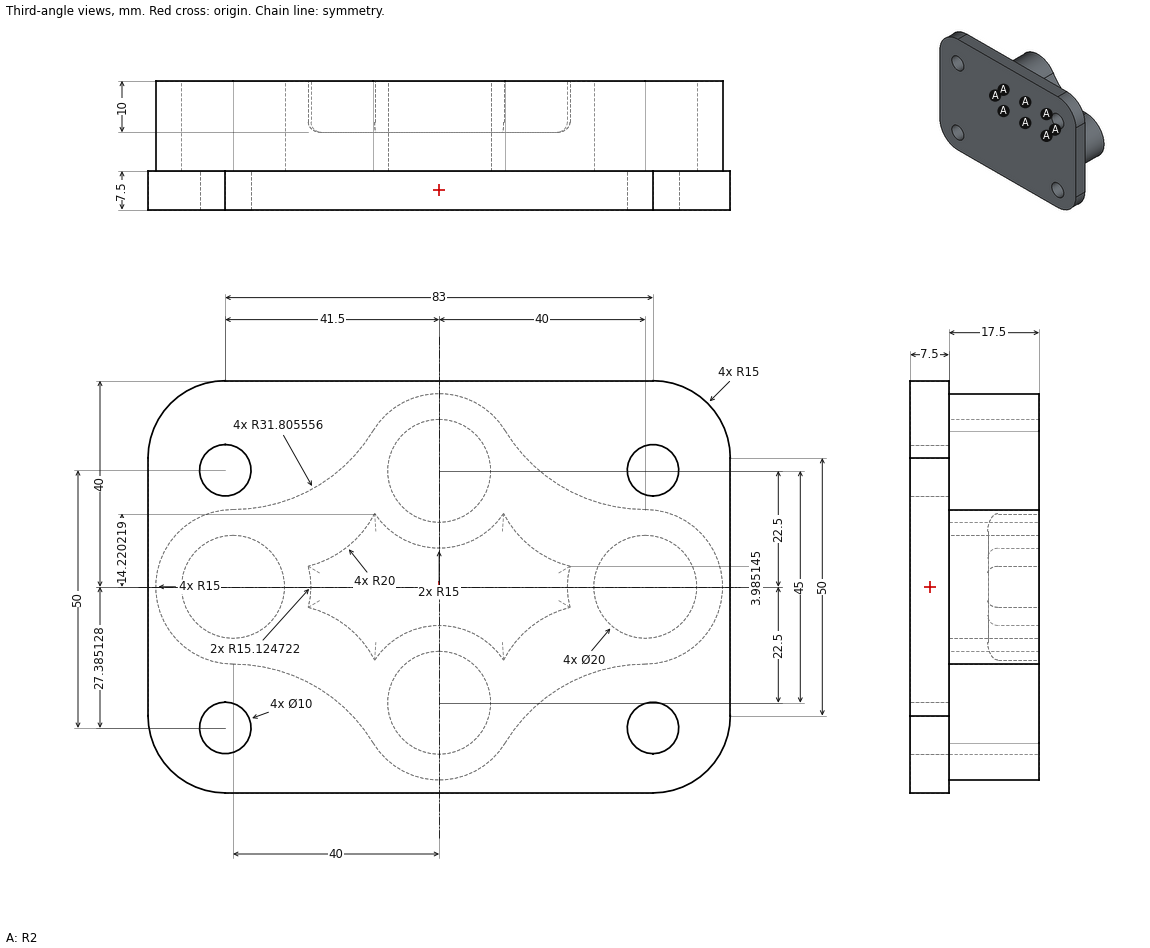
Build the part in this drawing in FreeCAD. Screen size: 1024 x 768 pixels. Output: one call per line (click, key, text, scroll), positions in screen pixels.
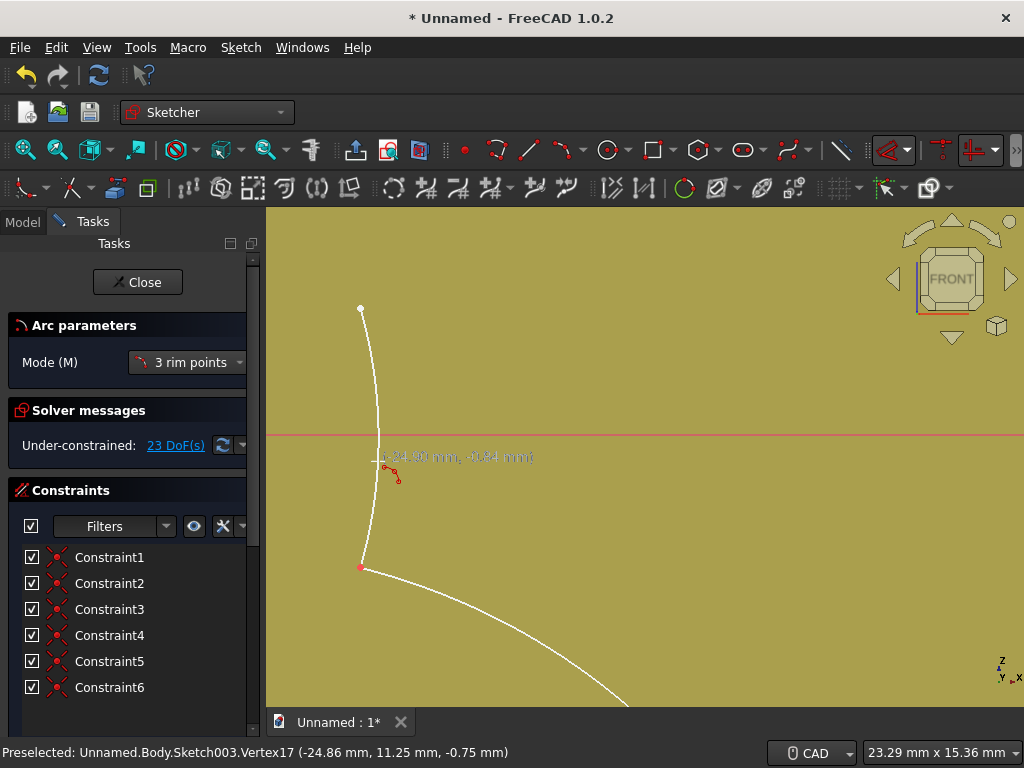
scroll(376, 464, down, 7)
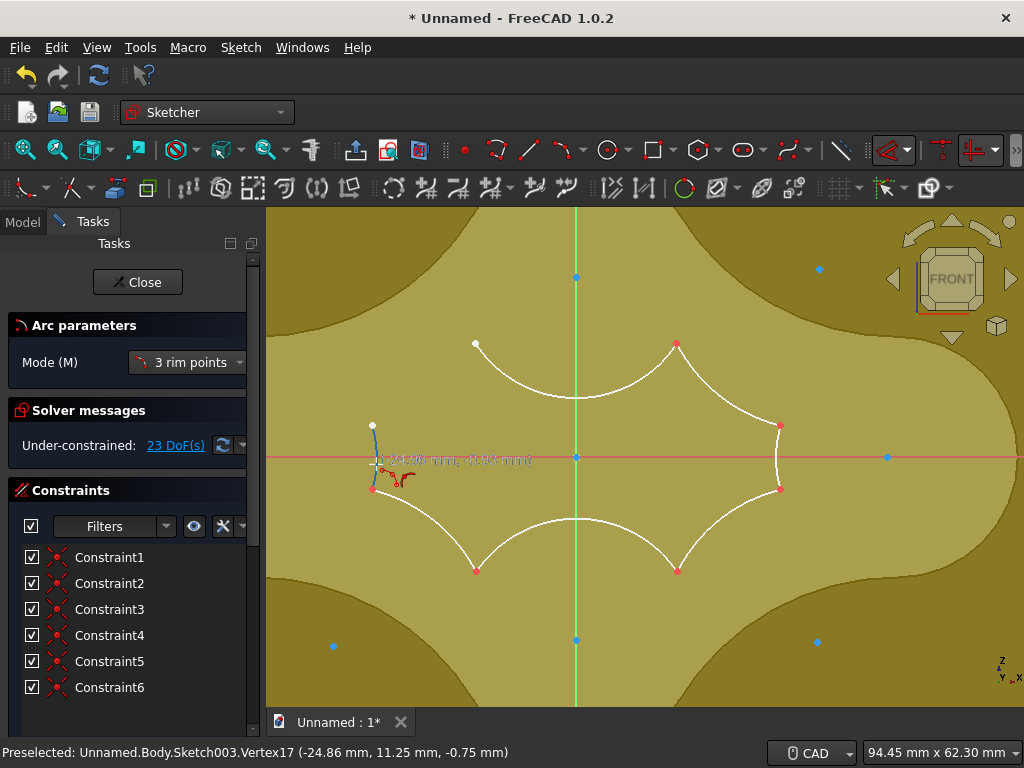
click(372, 426)
click(476, 344)
click(433, 395)
key(Escape)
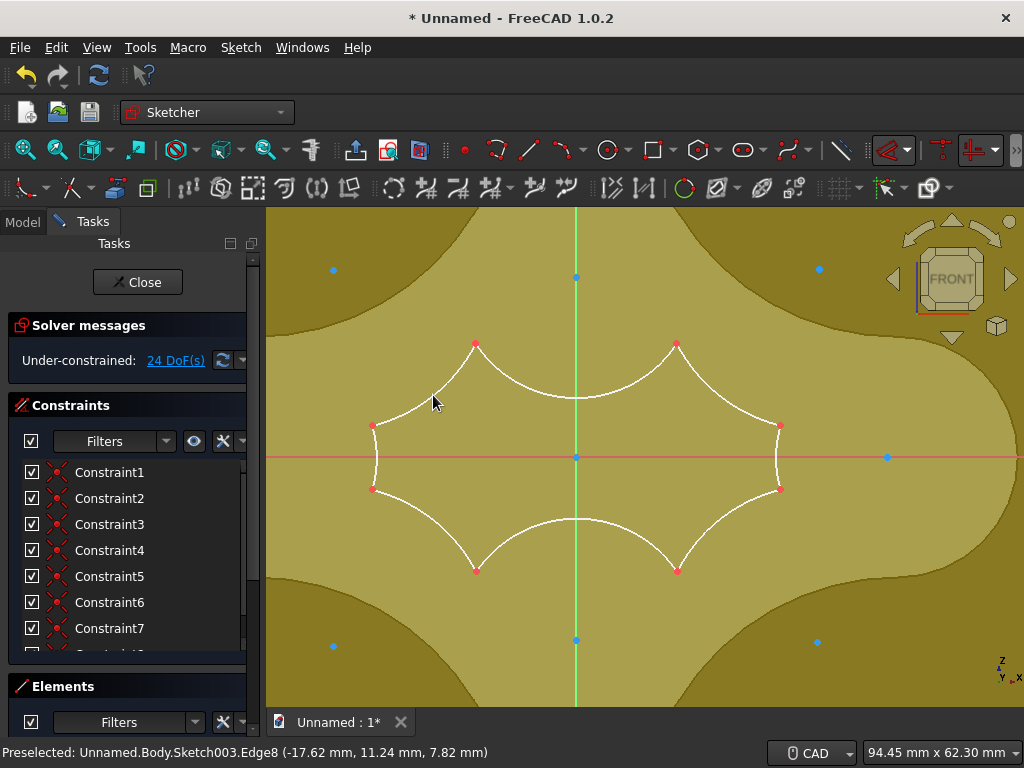
click(700, 377)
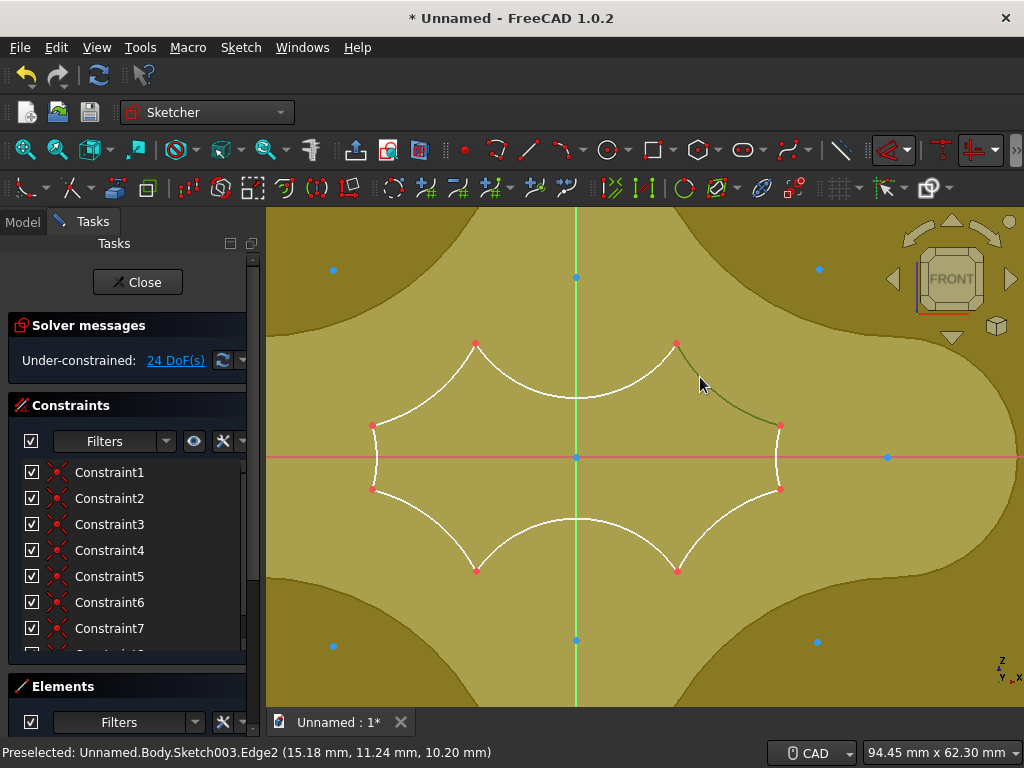
click(743, 504)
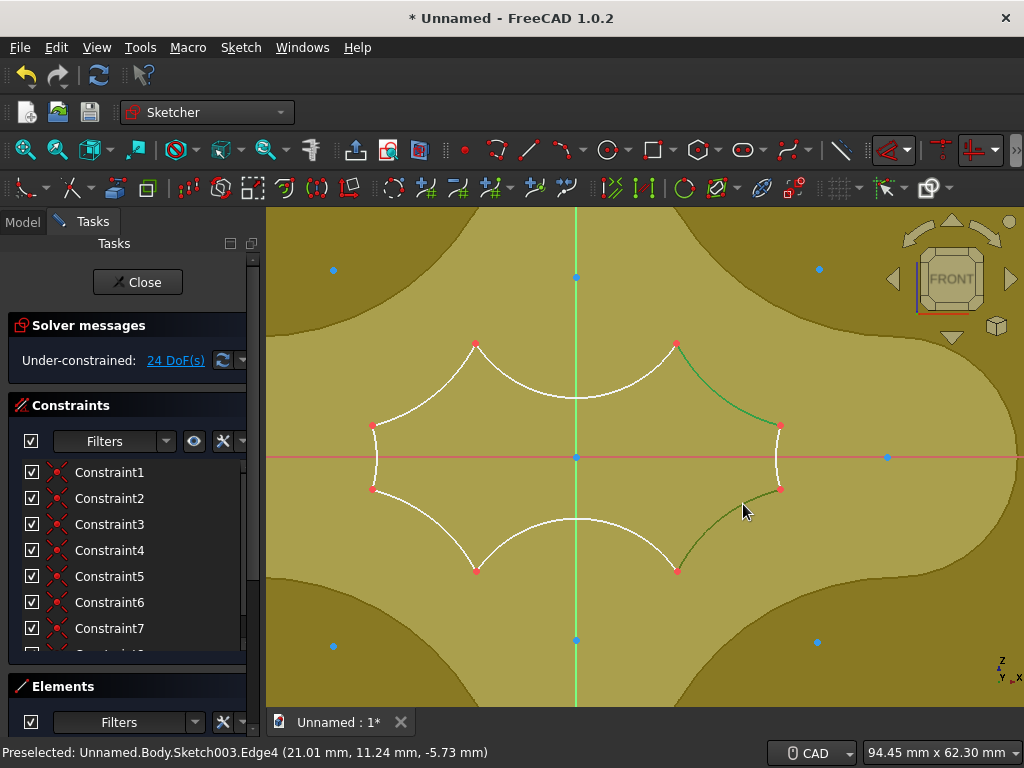
click(453, 538)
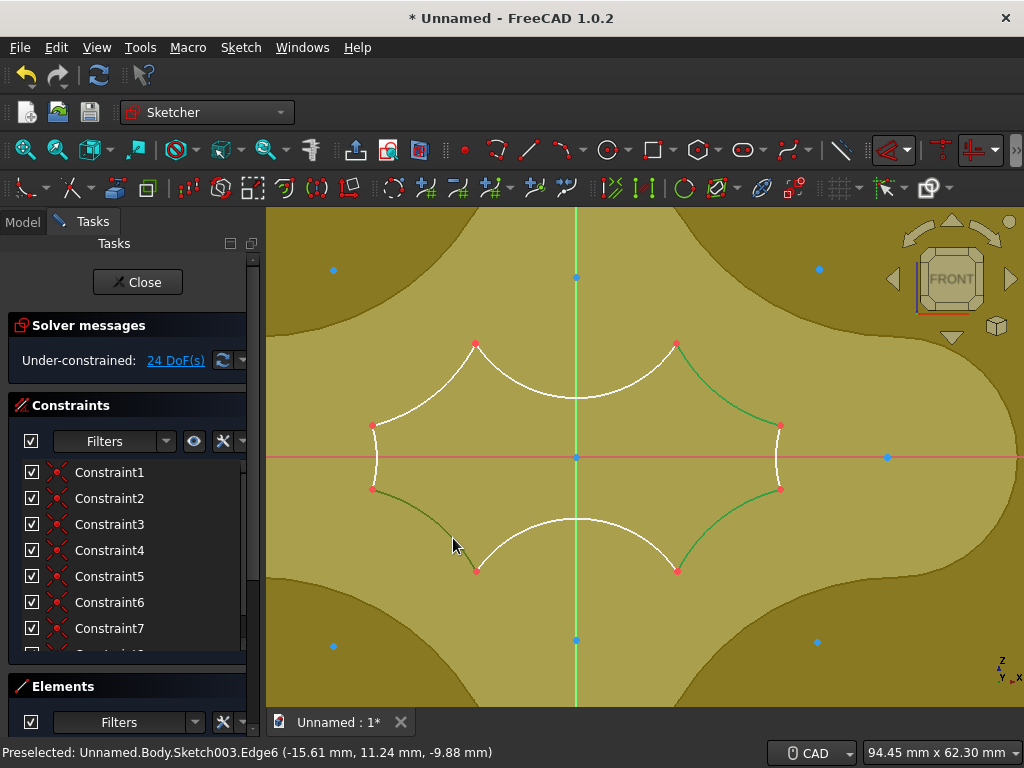
click(410, 411)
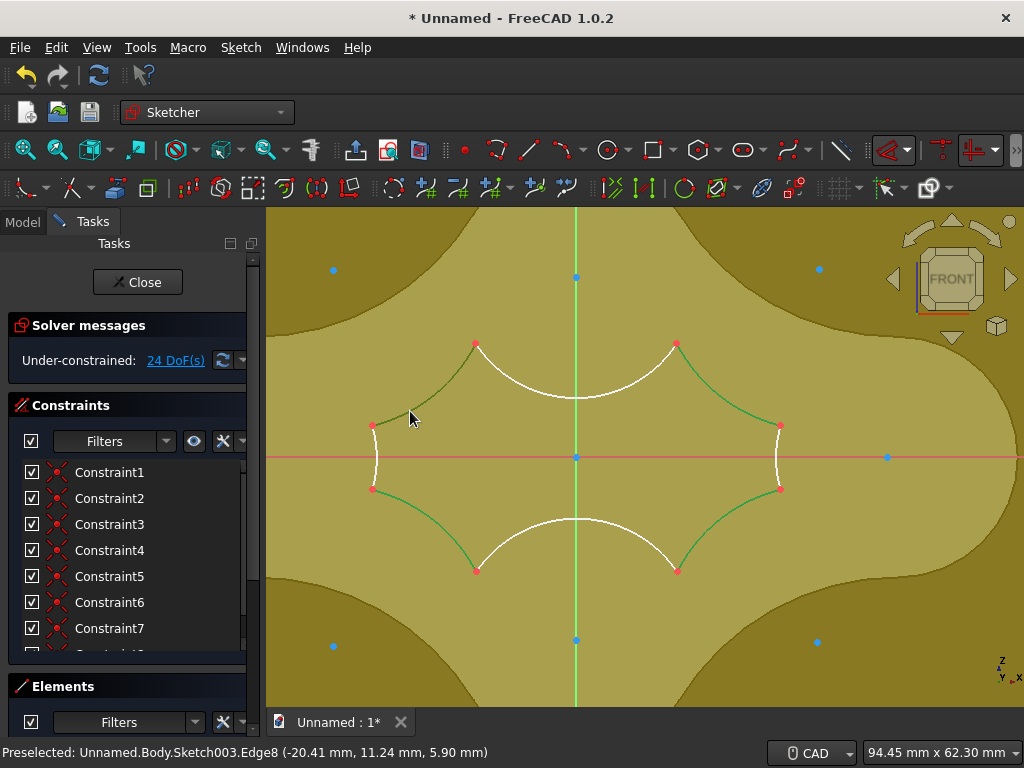
key(e)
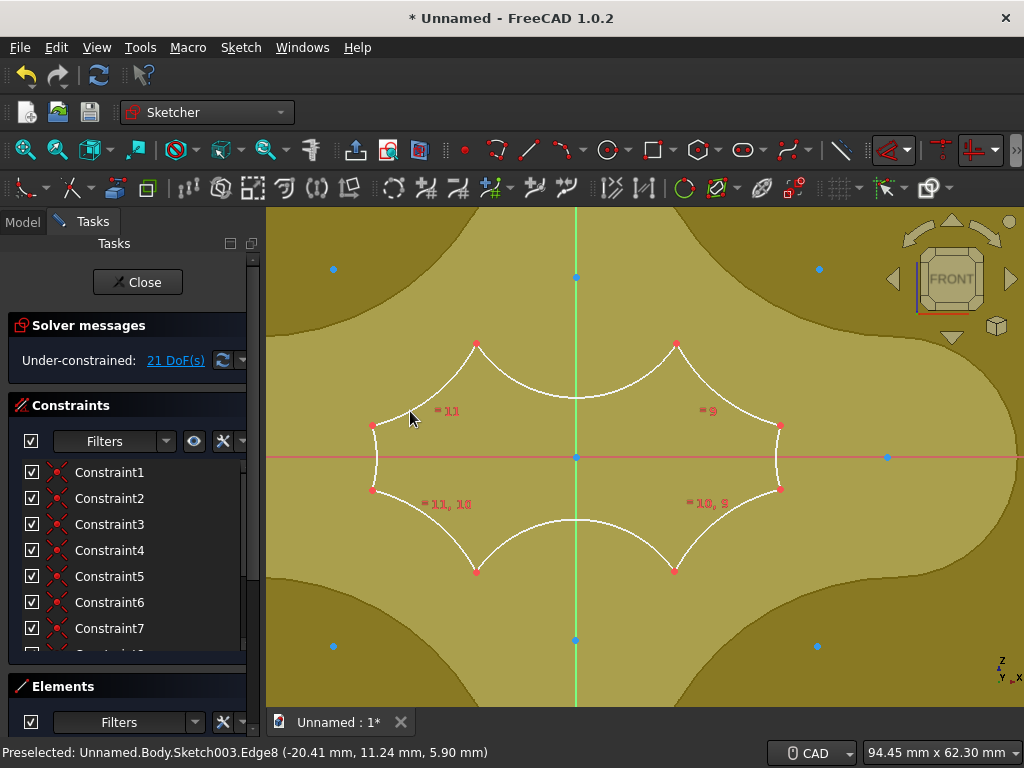
click(530, 389)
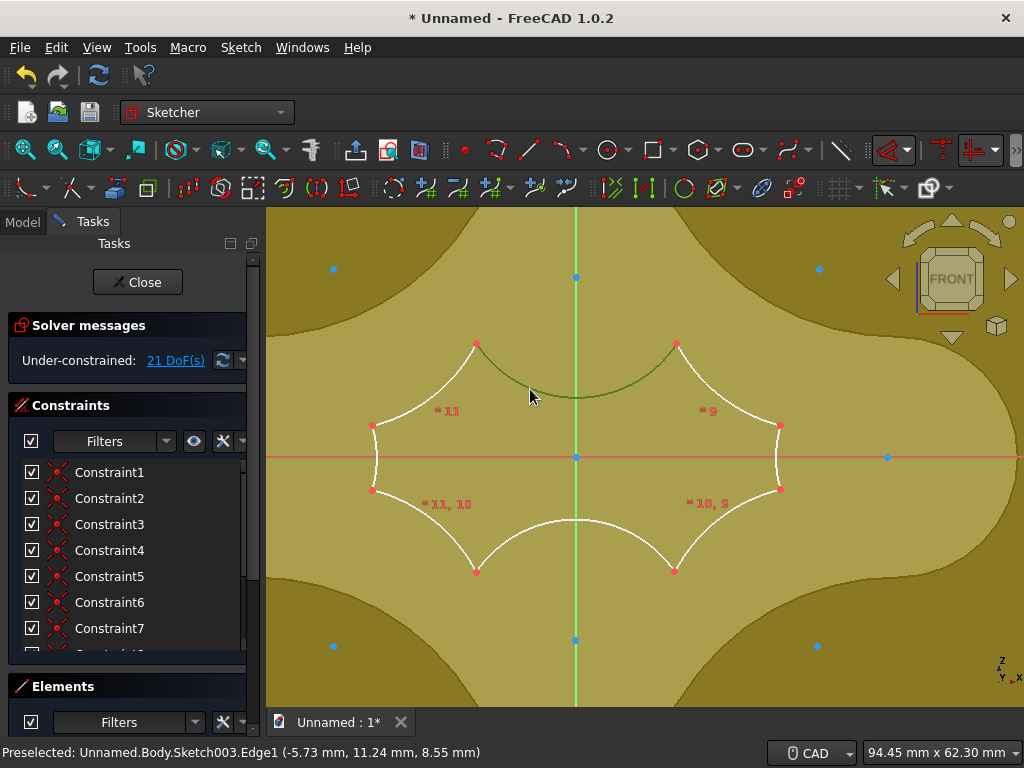
click(621, 529)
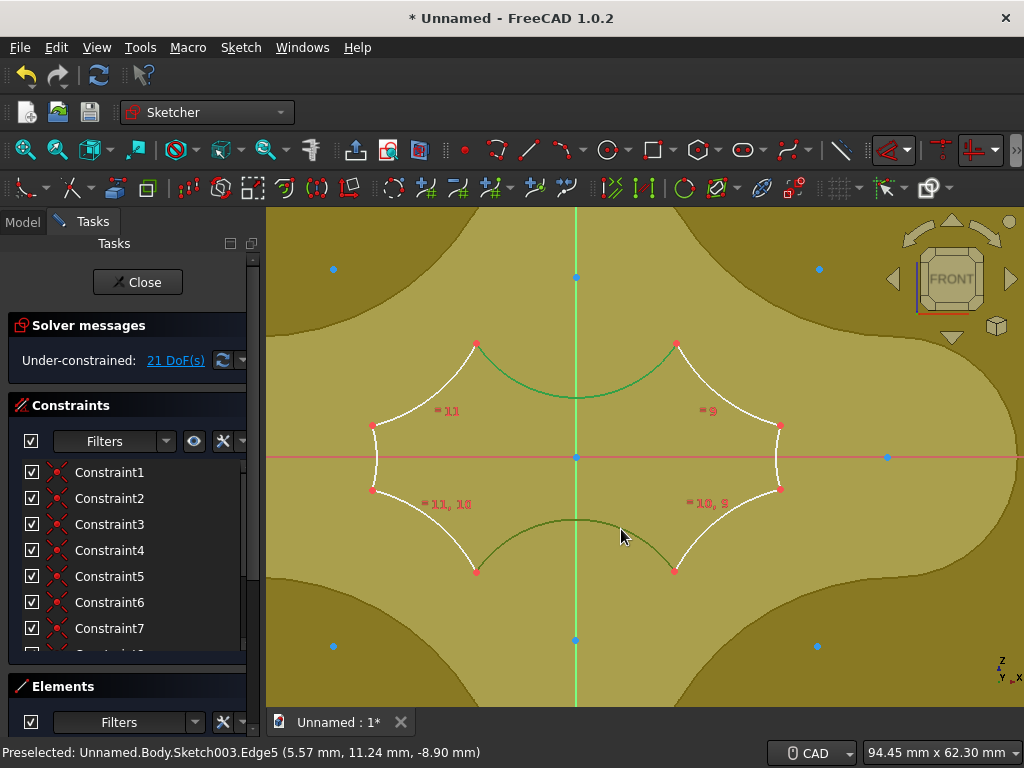
key(e)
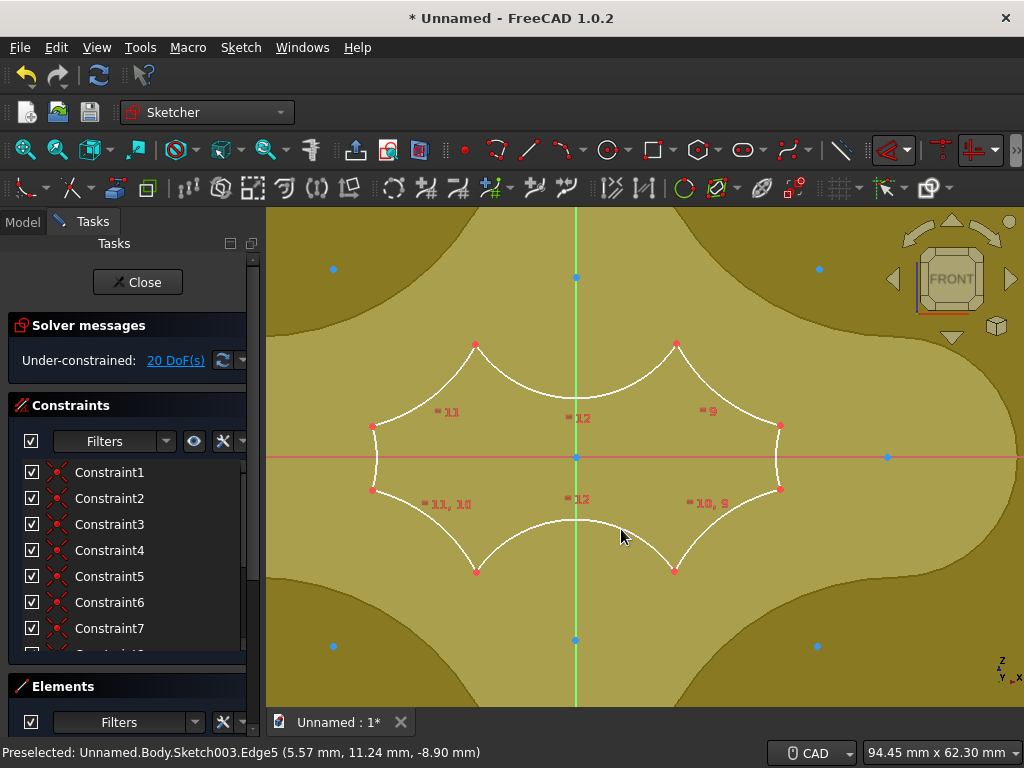
click(777, 445)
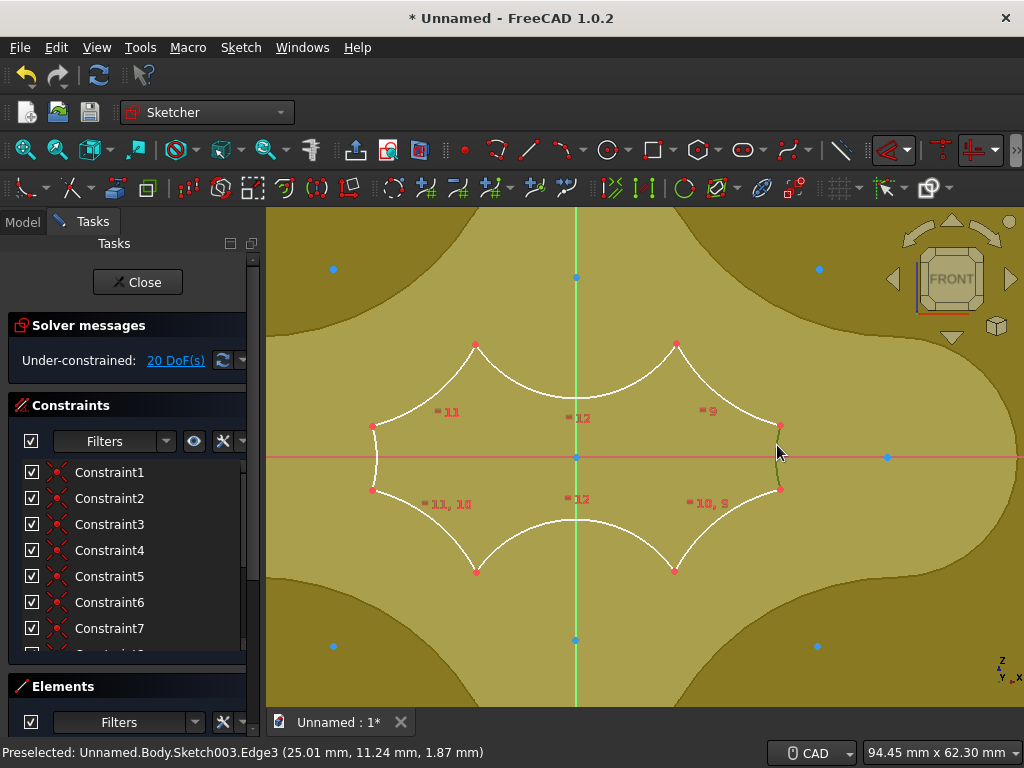
click(376, 471)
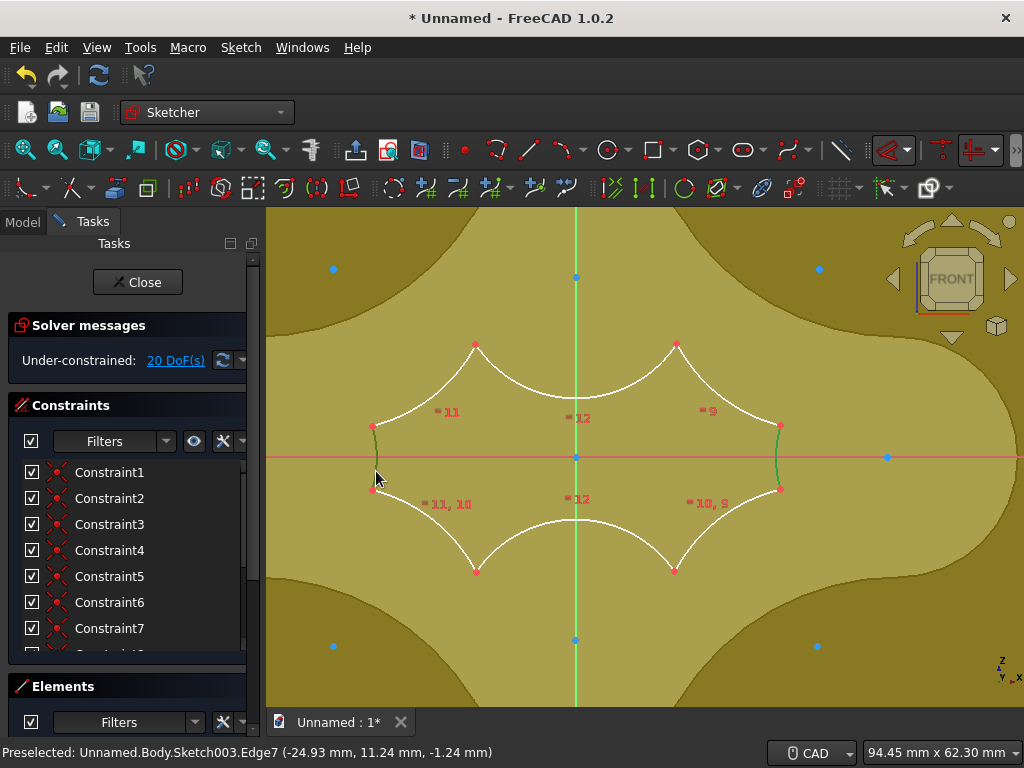
key(e)